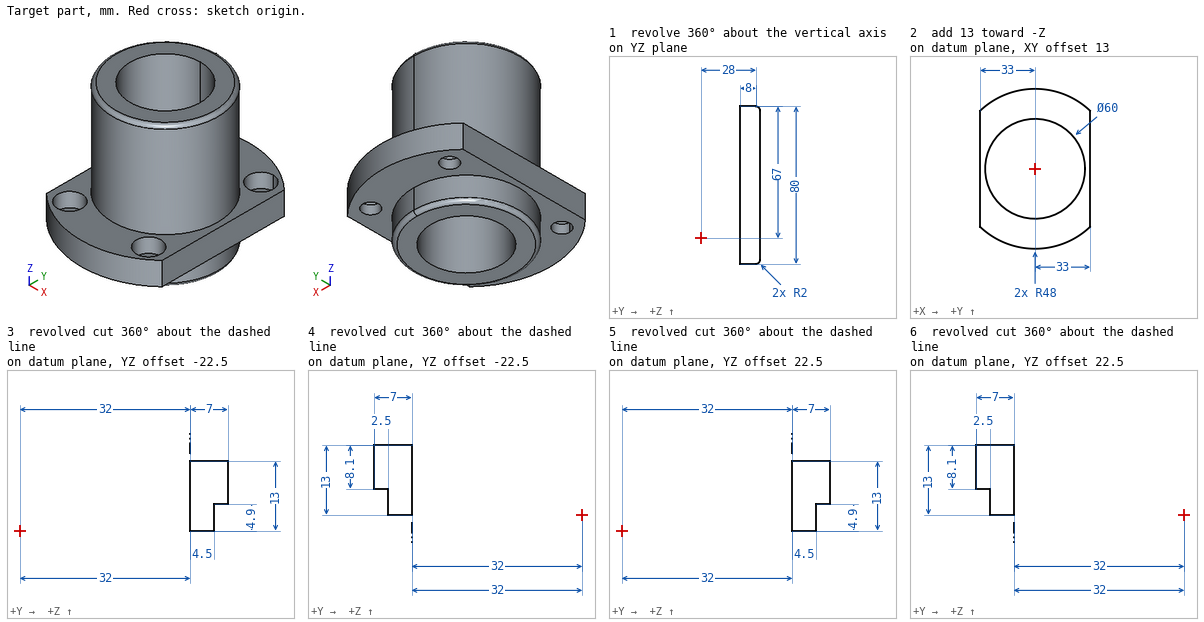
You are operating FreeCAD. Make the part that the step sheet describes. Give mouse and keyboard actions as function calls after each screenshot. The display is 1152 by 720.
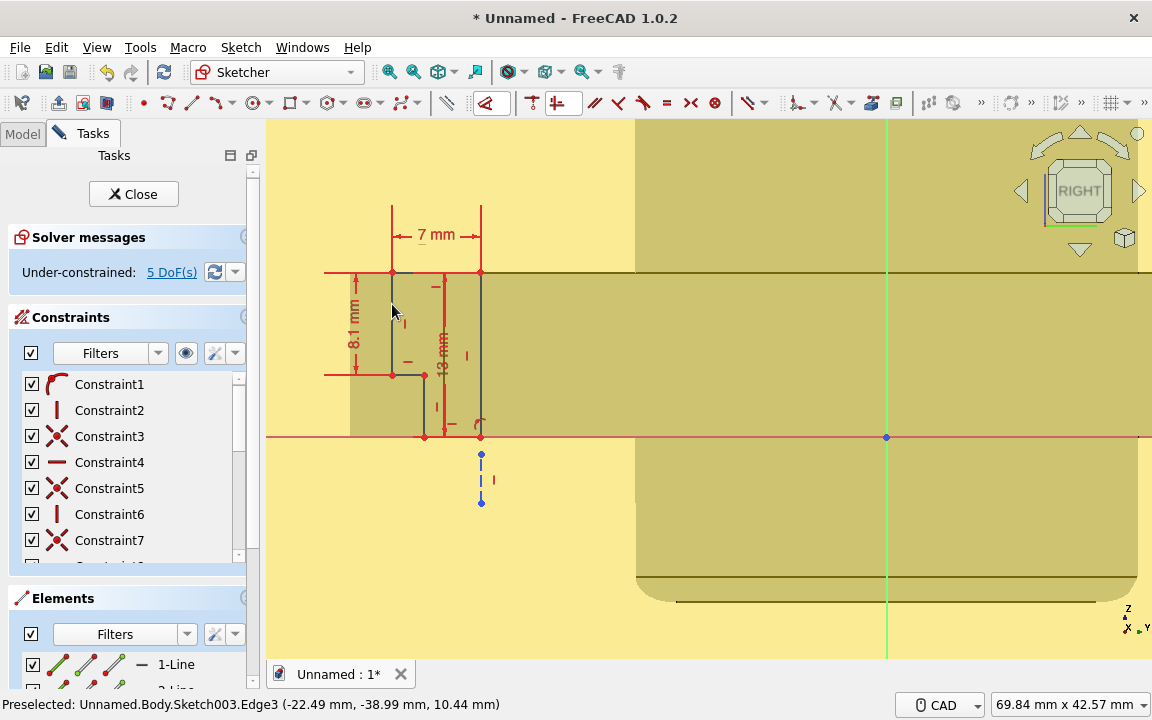
scroll(402, 375, up, 2)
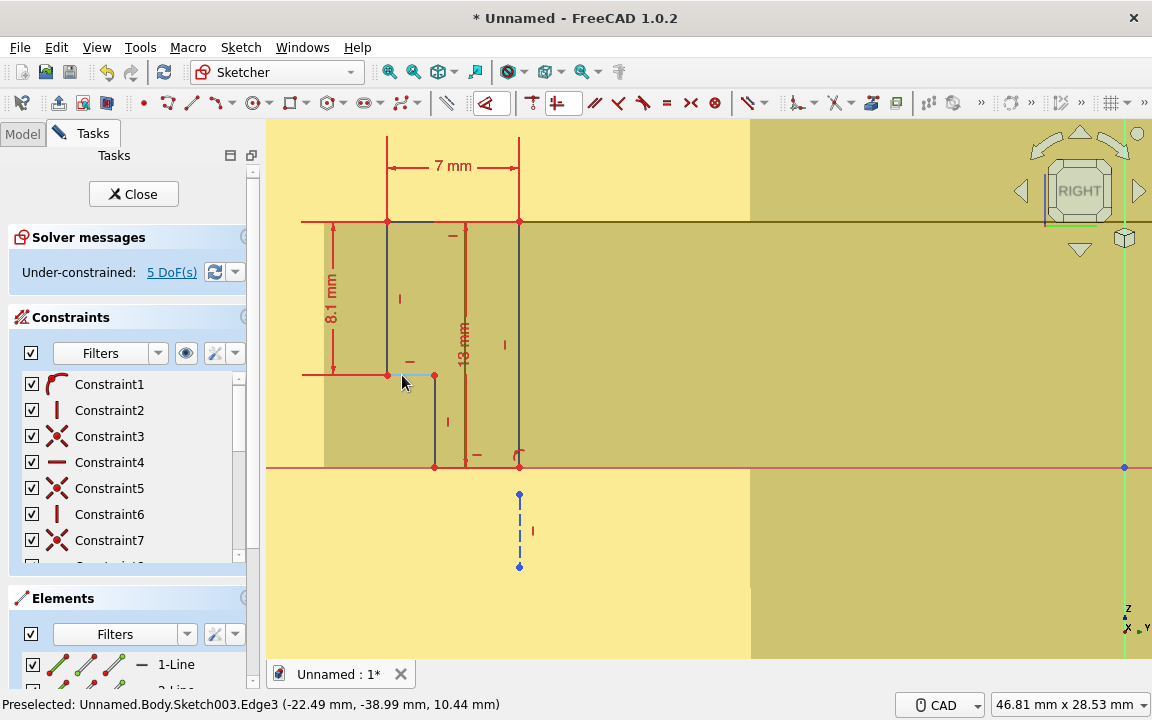
click(401, 375)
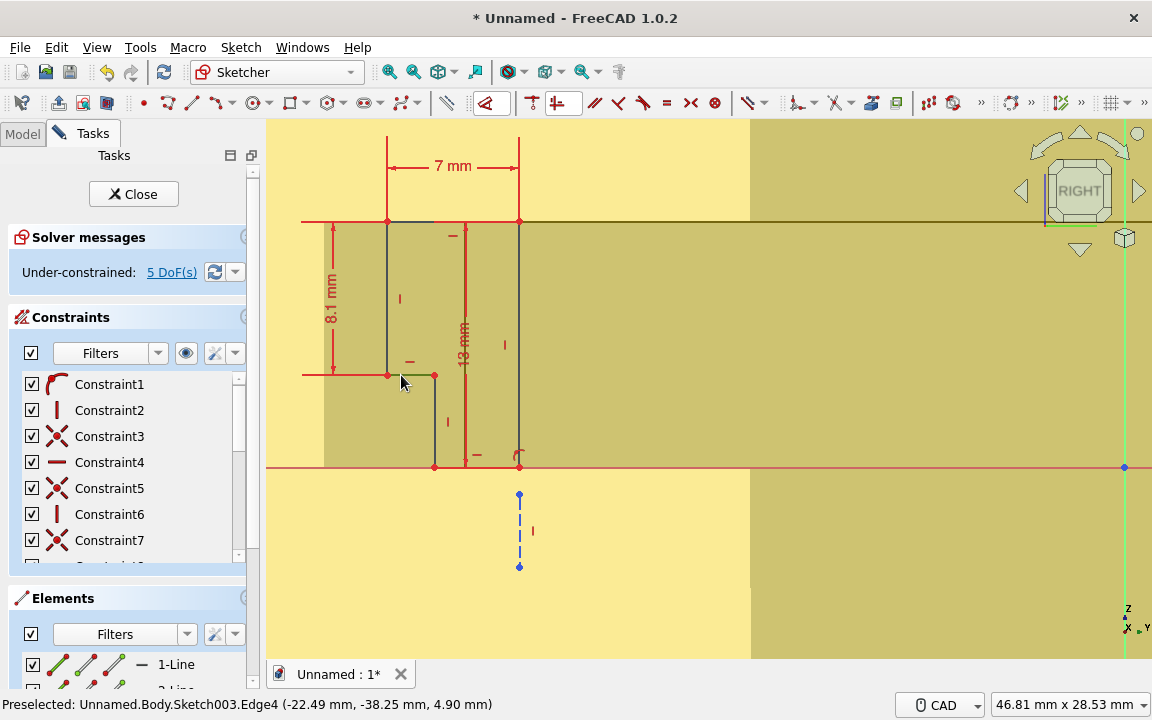
key(l)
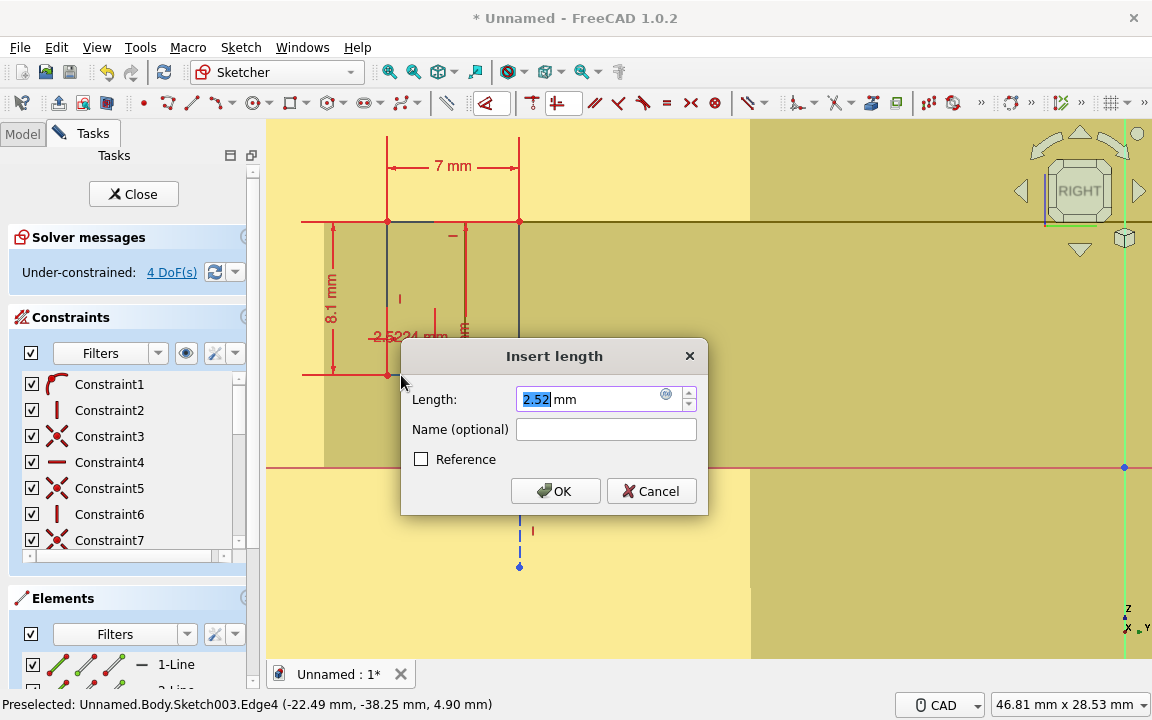
text(2.5)
key(Return)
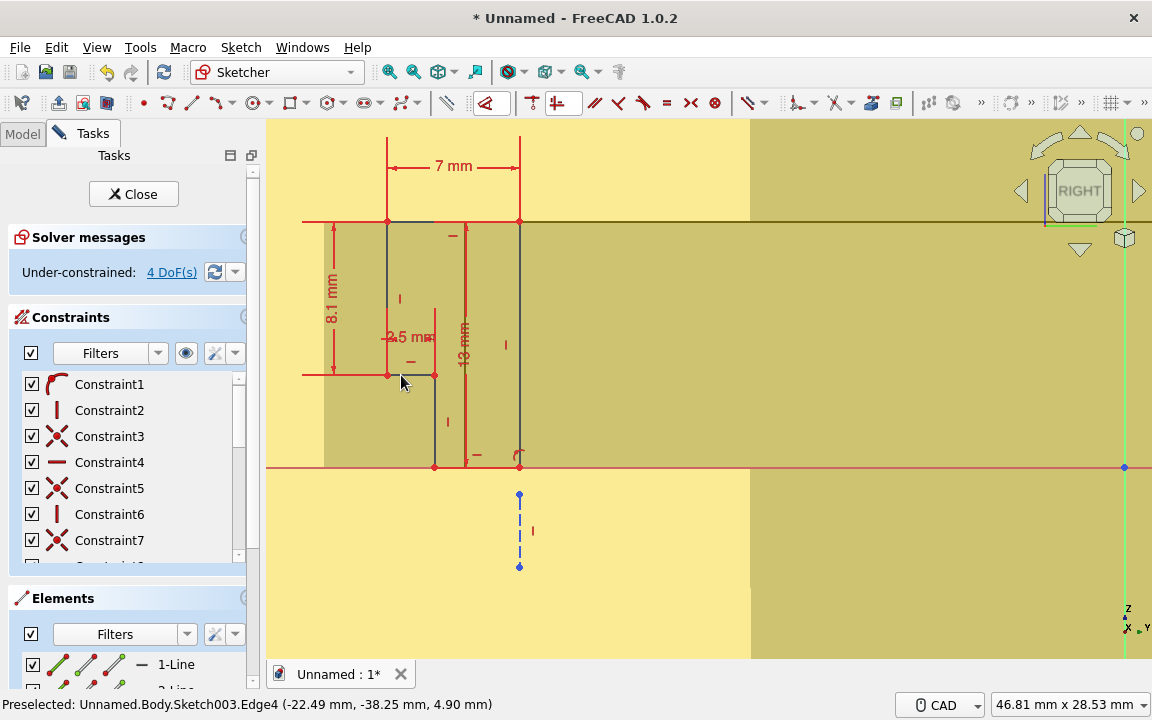
click(520, 468)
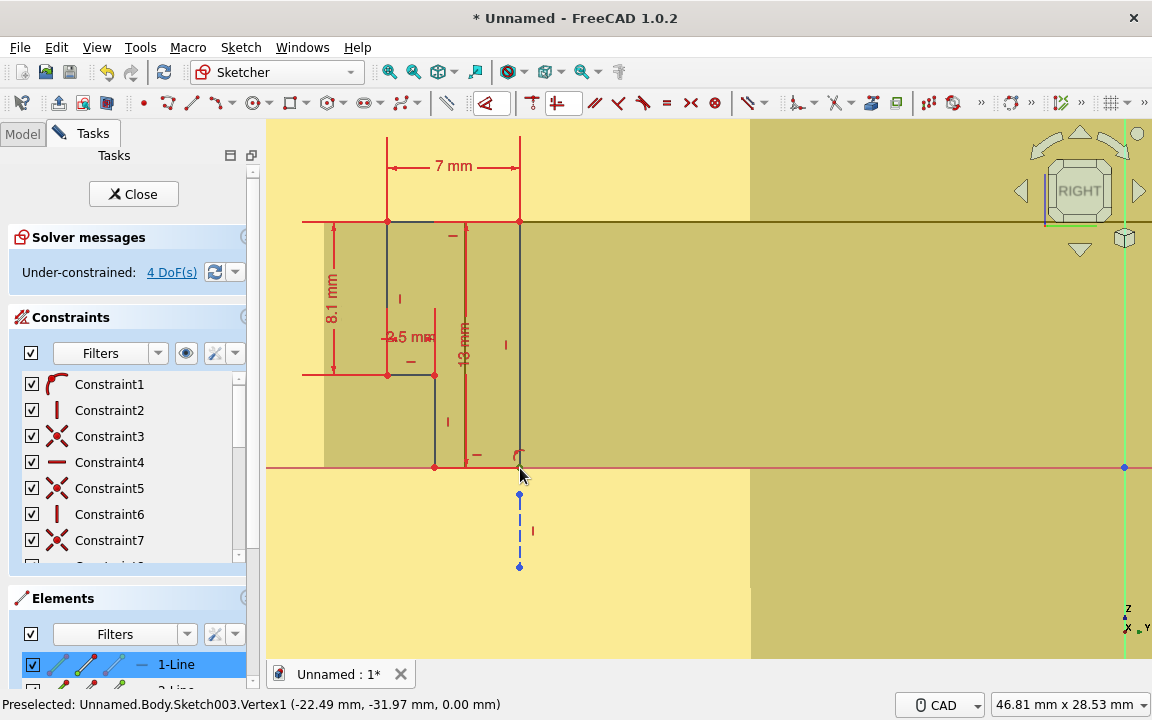
key(l)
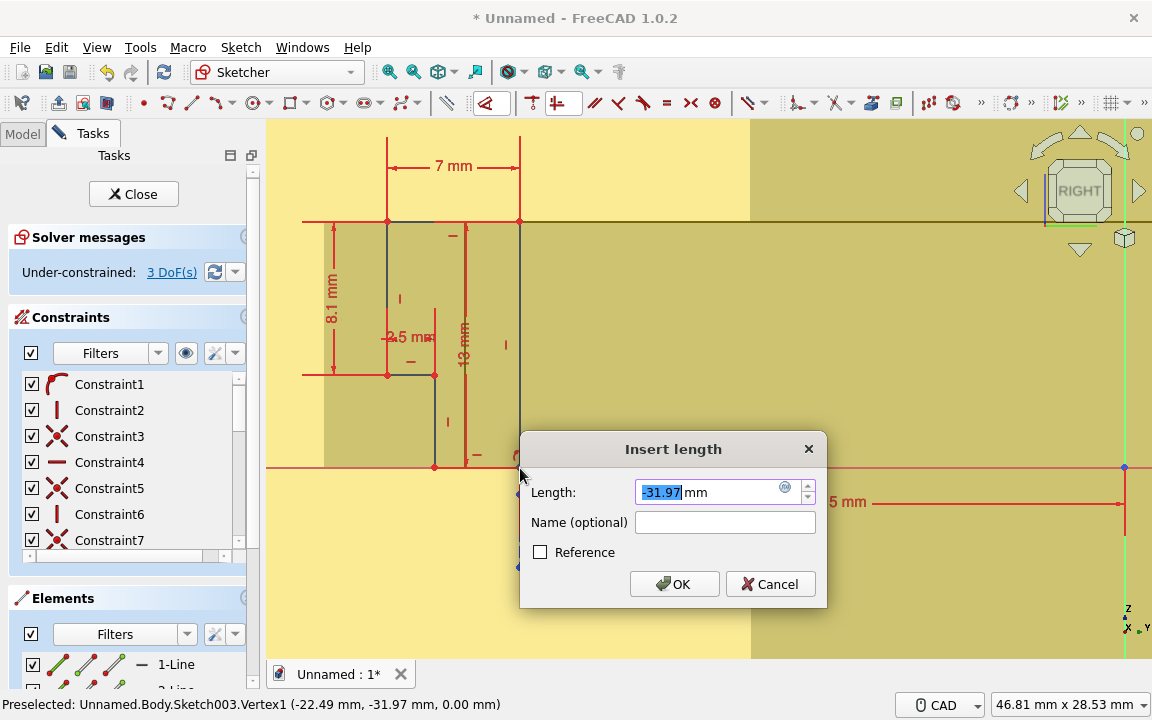
text(-32)
key(Return)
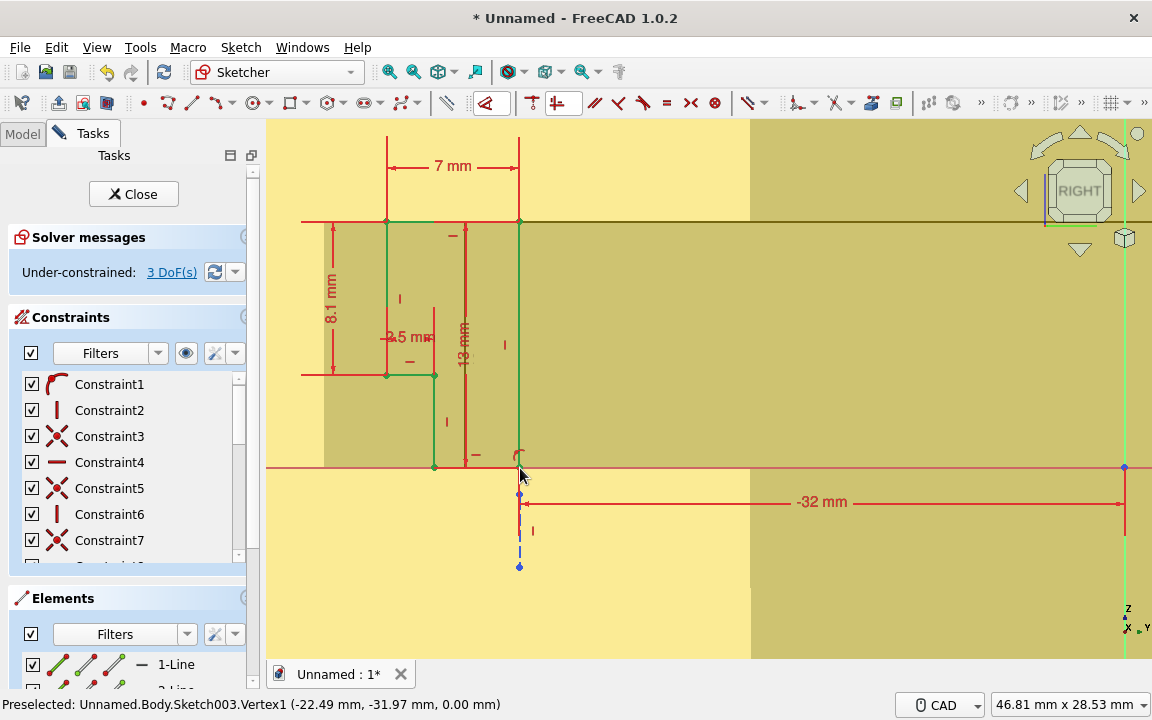
click(520, 494)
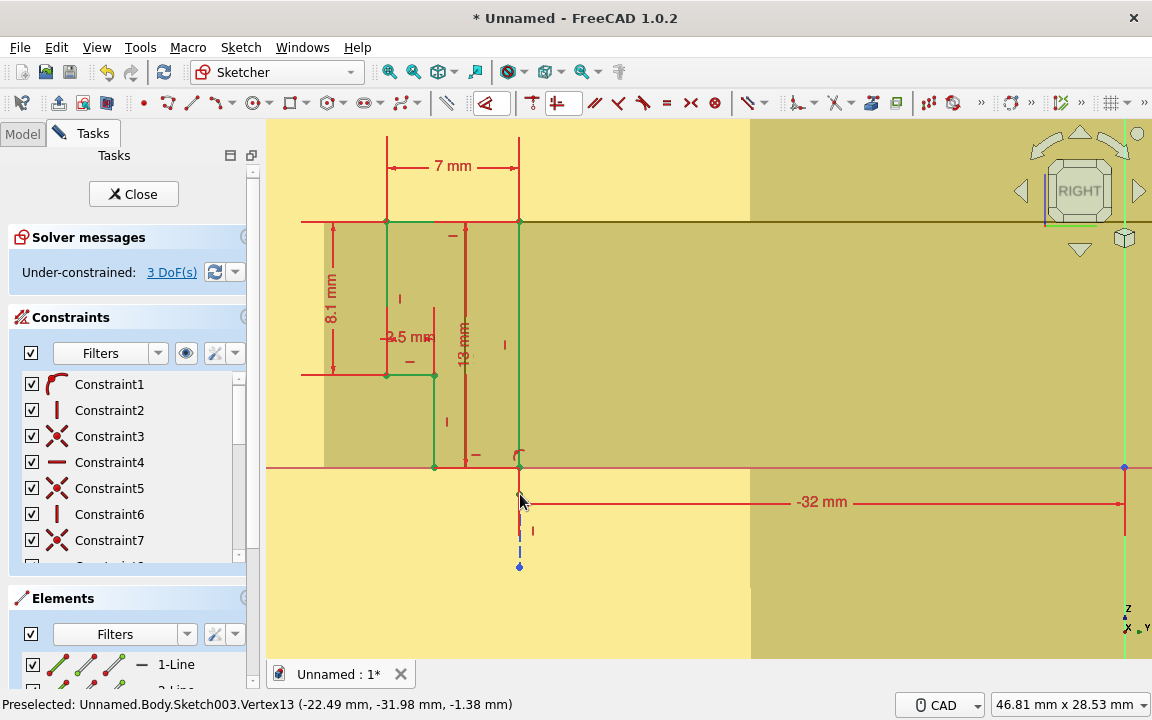
key(l)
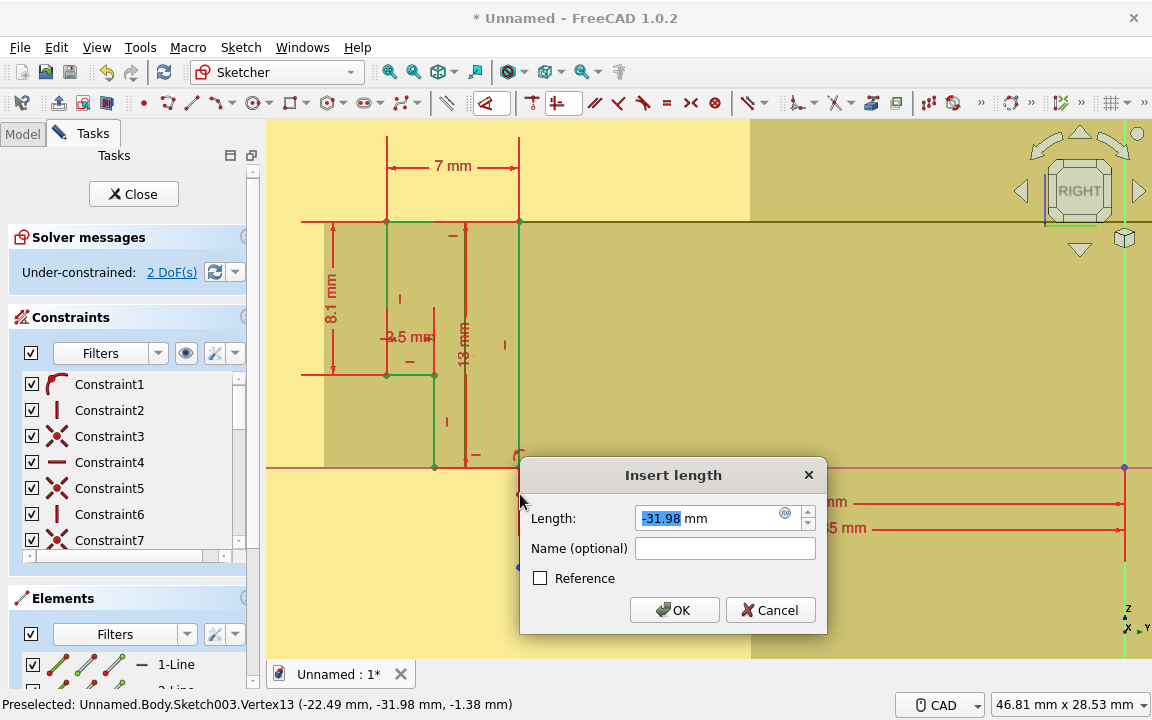
text(-32)
key(Return)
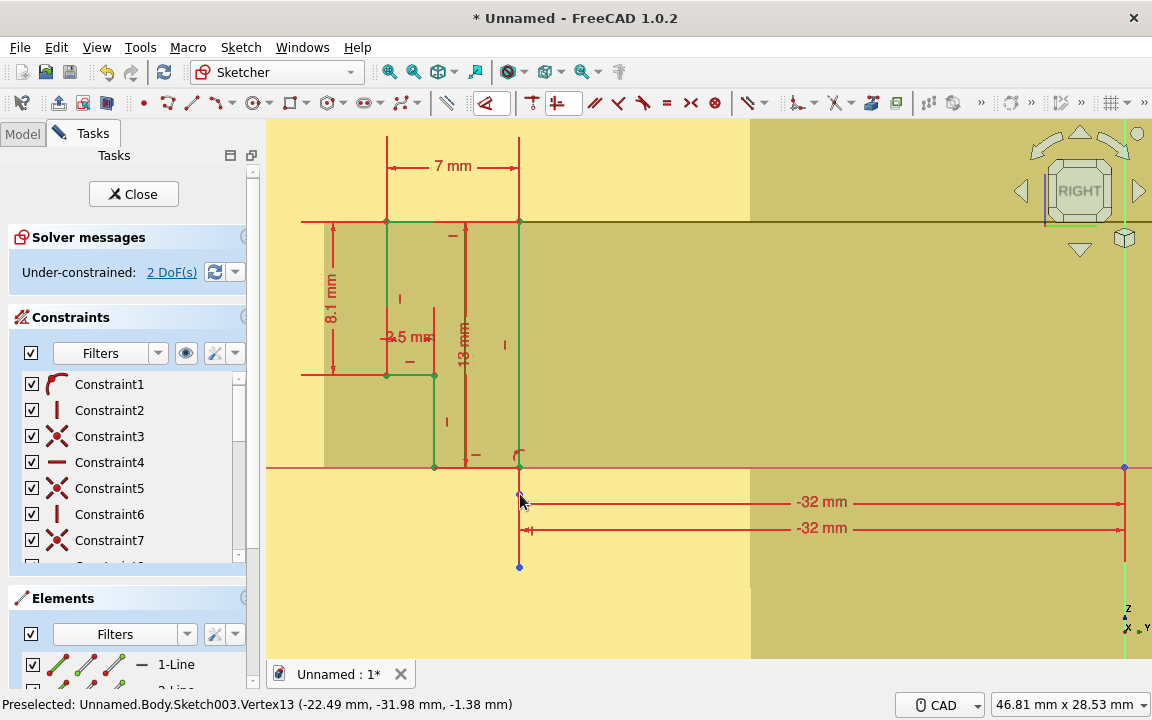
click(134, 194)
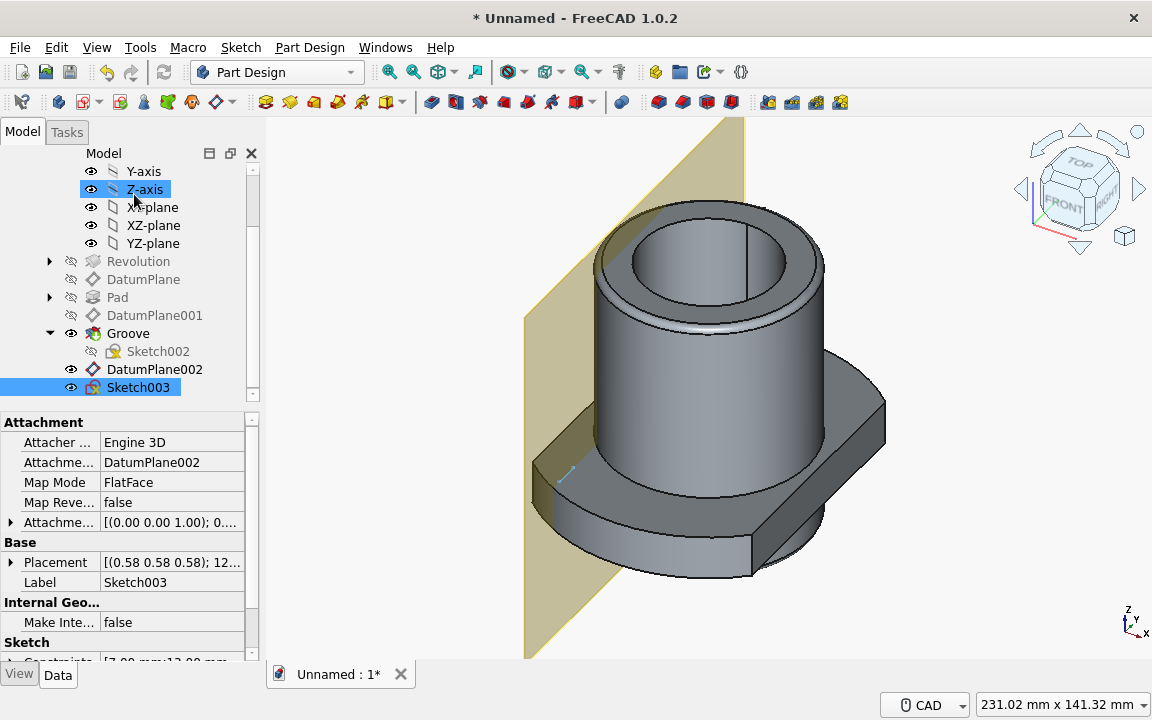
click(480, 102)